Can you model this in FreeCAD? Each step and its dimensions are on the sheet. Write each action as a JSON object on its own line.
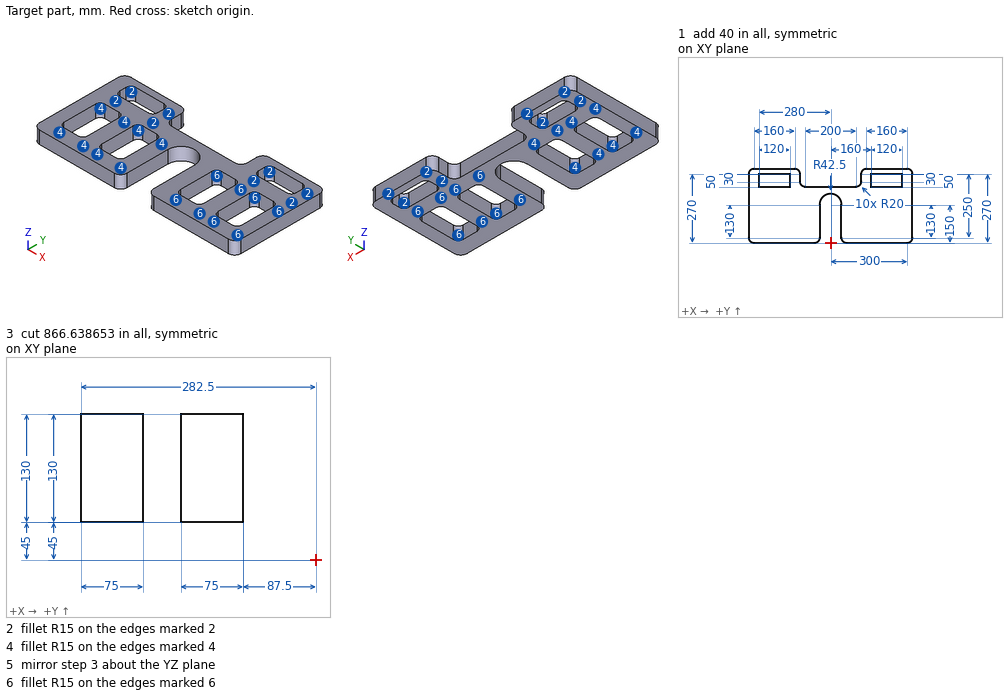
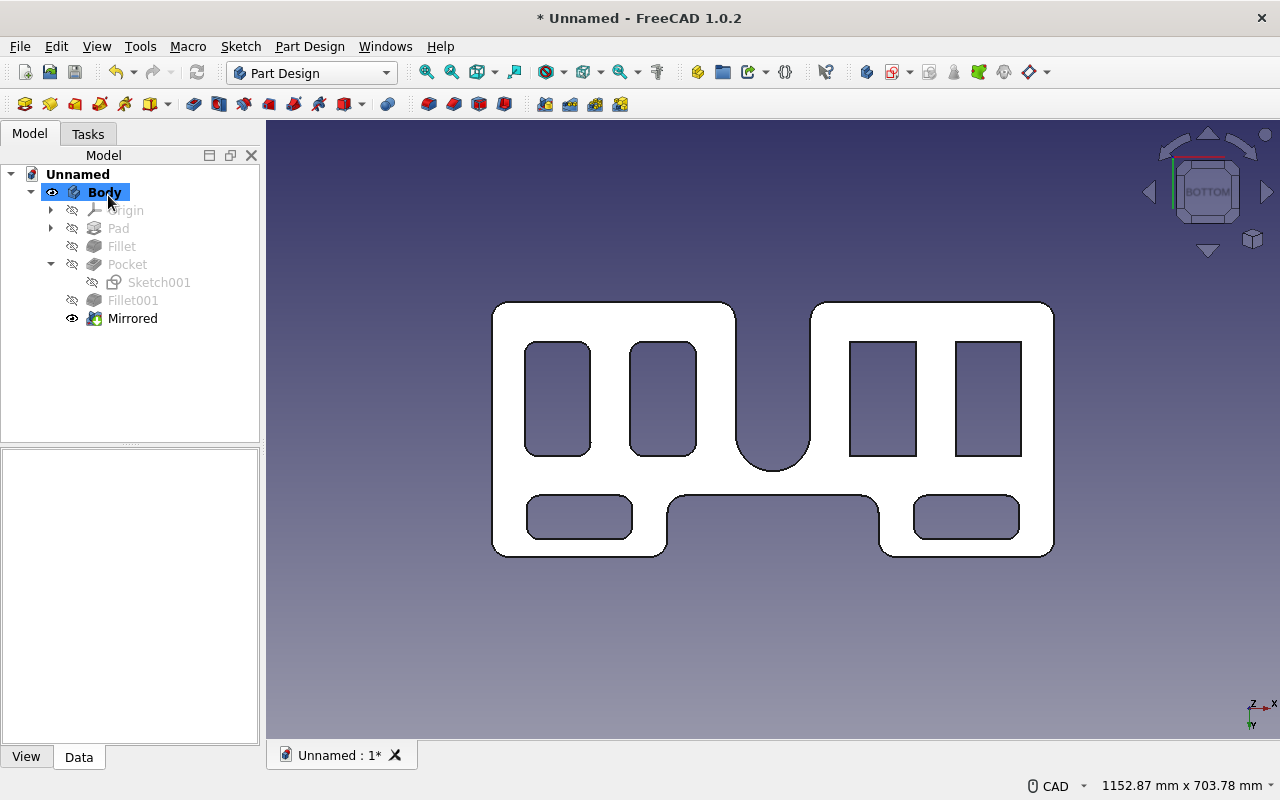
{"action": "key", "text": "4"}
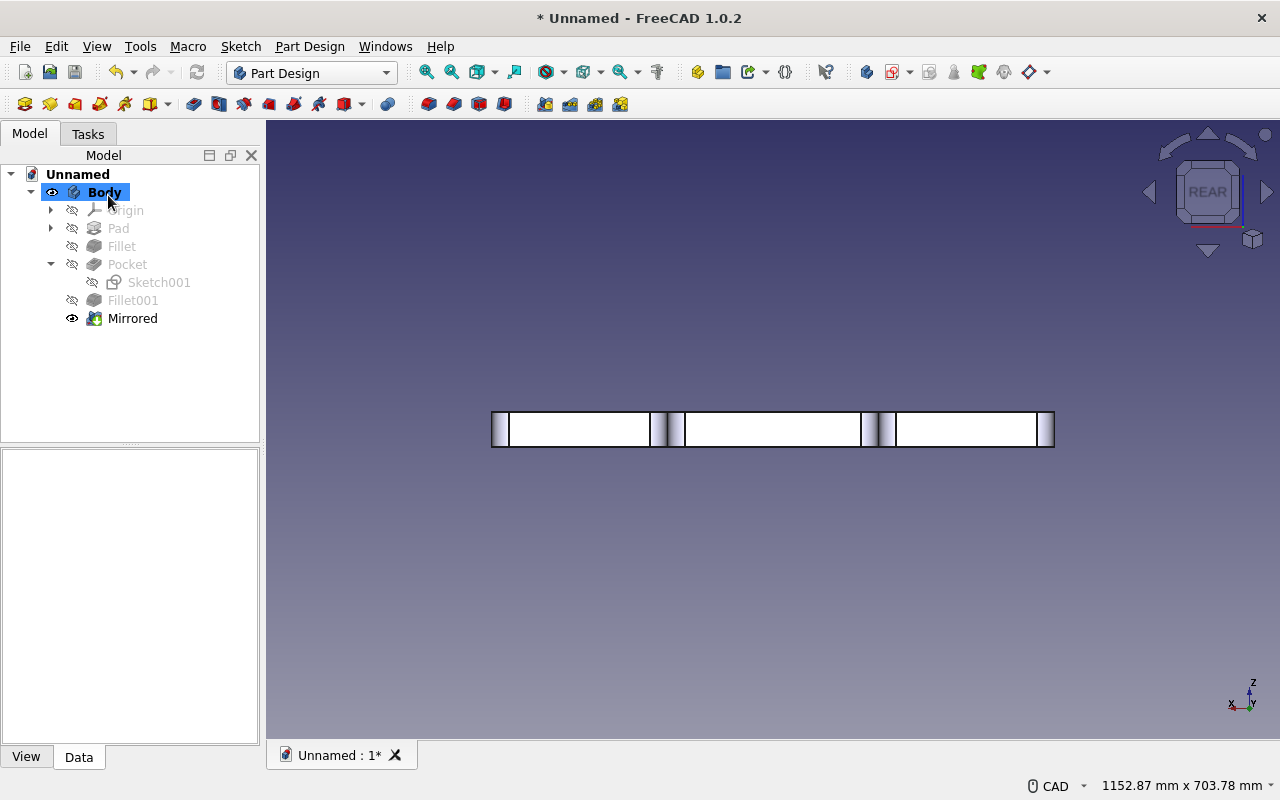
{"action": "key", "text": "6"}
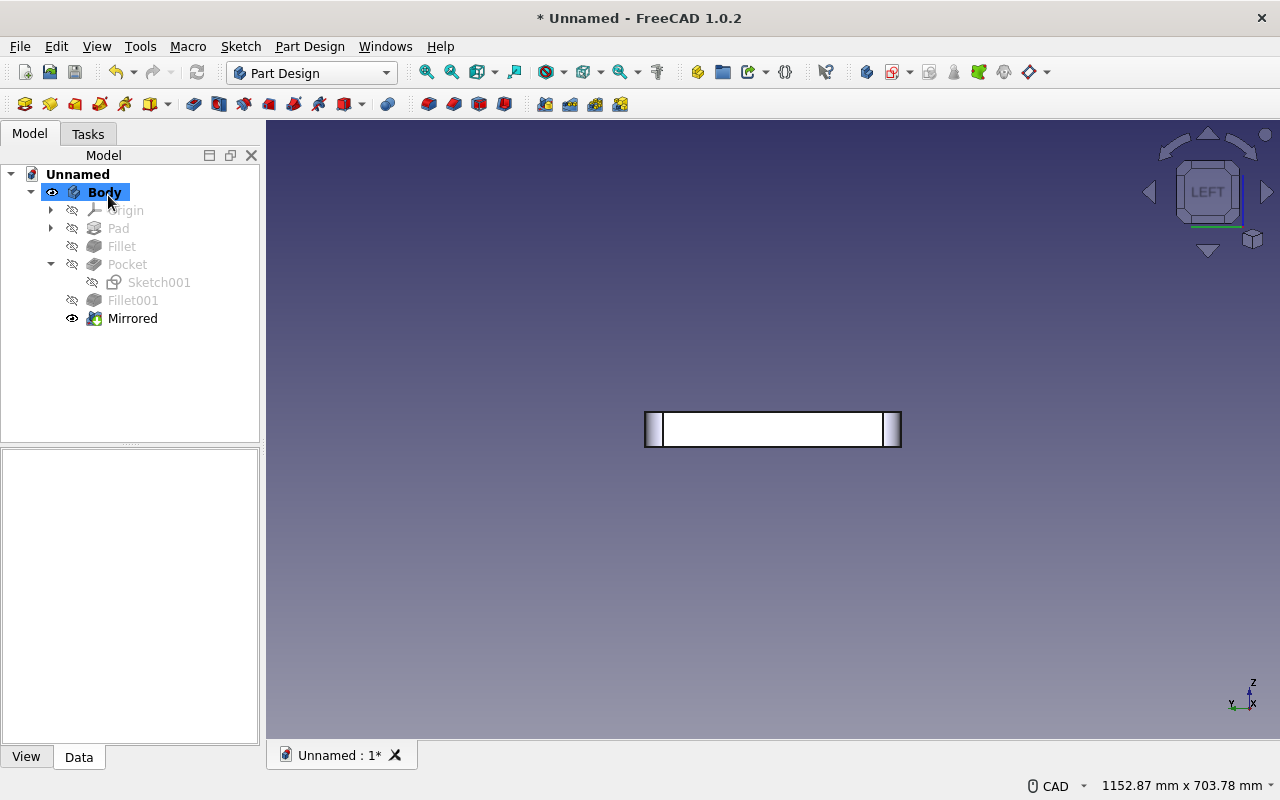
{"action": "left_click", "coordinate": [427, 72]}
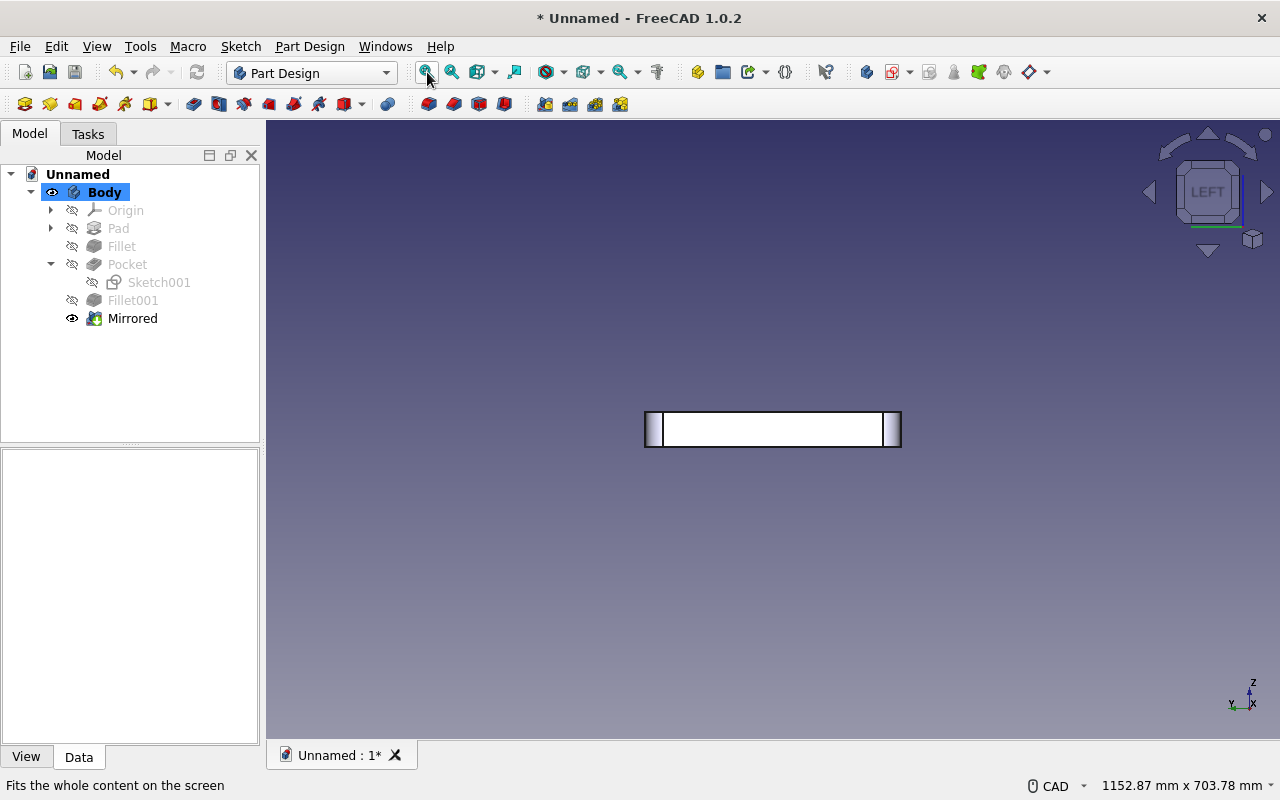
{"action": "key", "text": "v 3"}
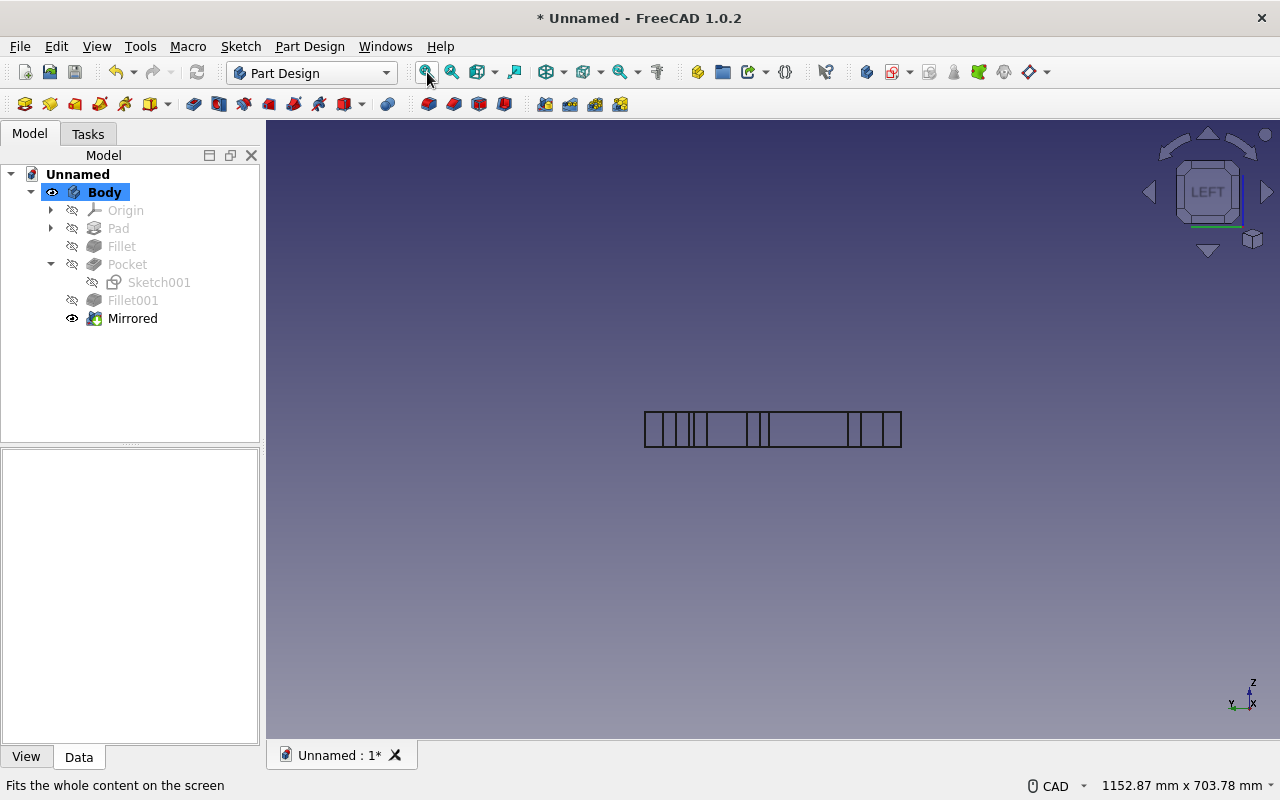
{"action": "key", "text": "0"}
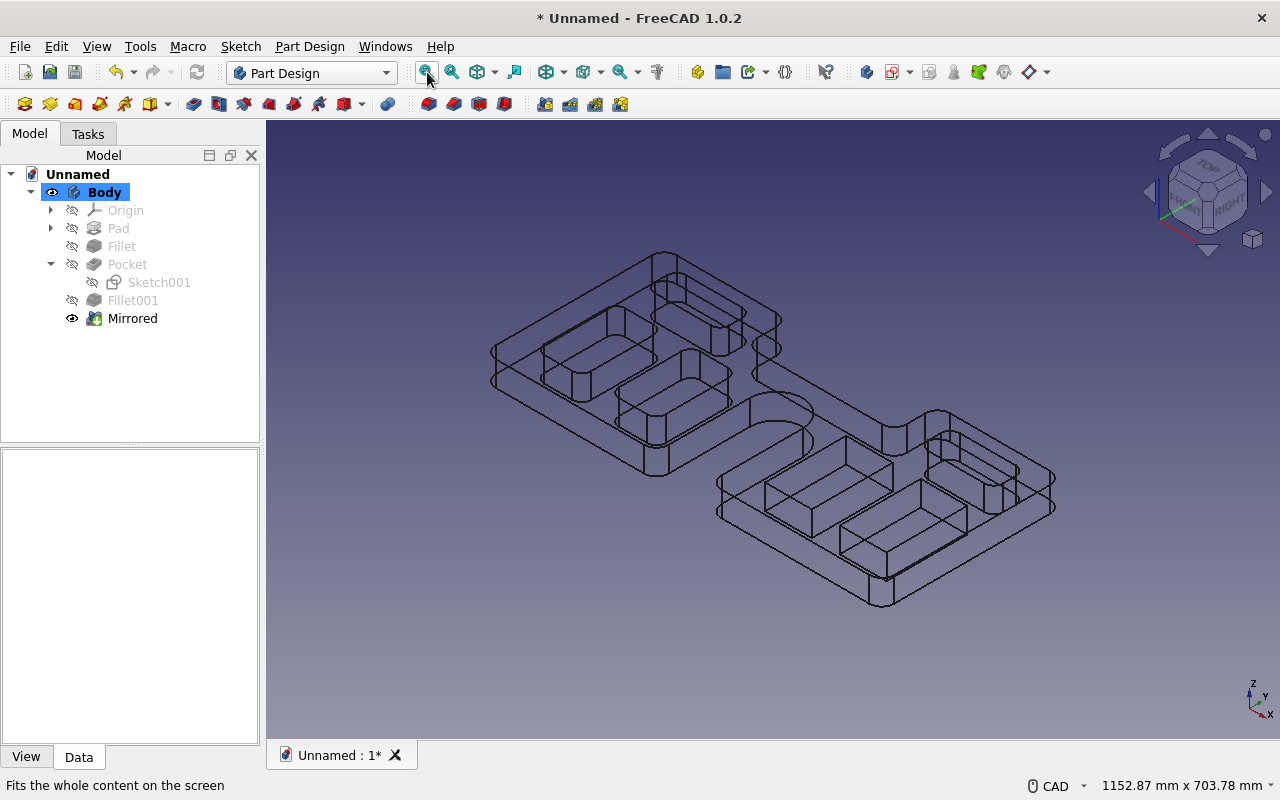
{"action": "left_click", "coordinate": [921, 492]}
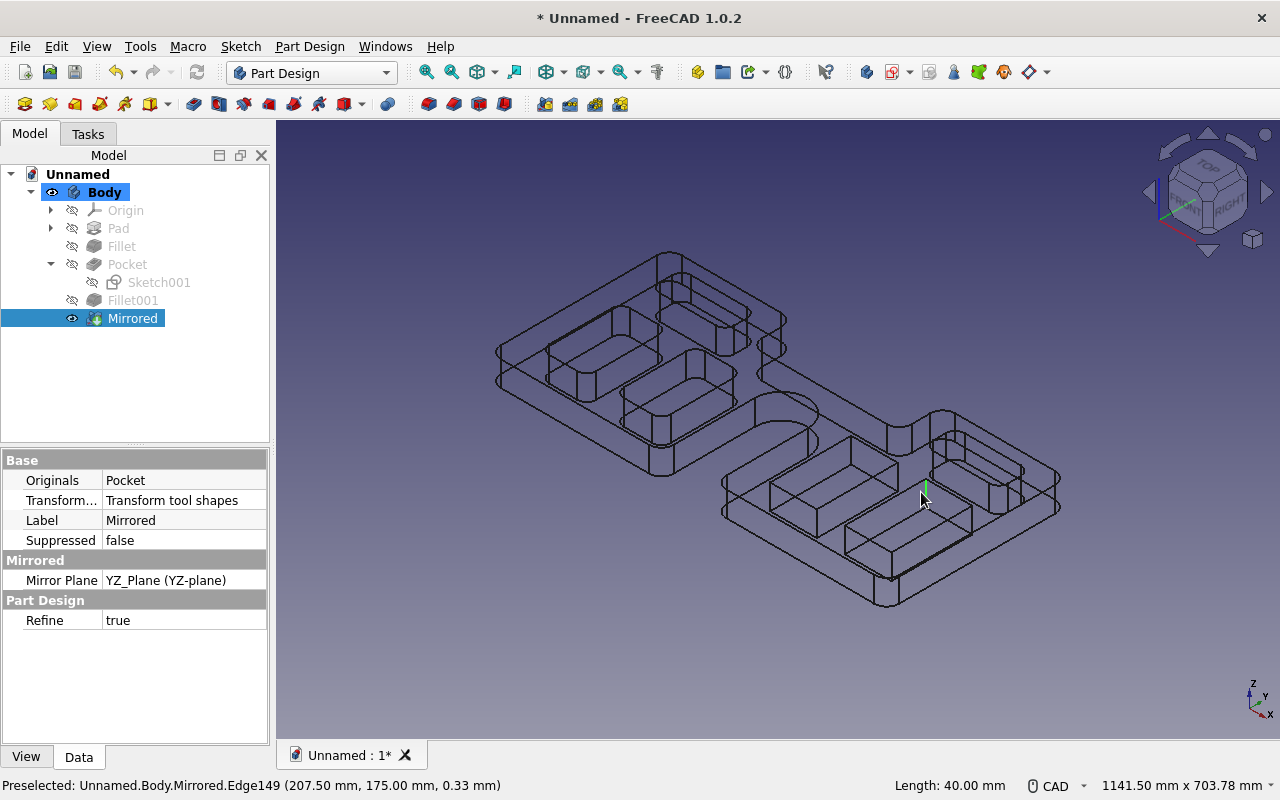
{"action": "left_click", "coordinate": [845, 539], "text": "ctrl"}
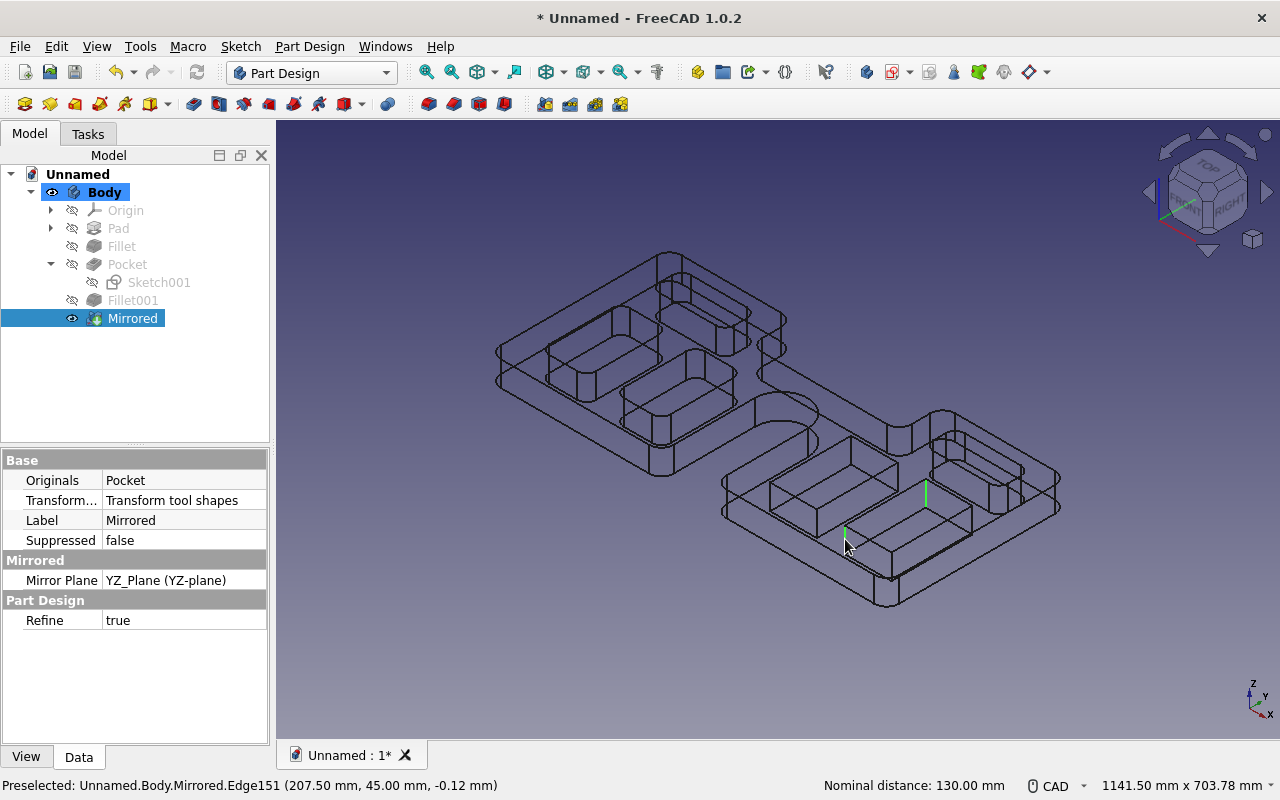
{"action": "left_click", "coordinate": [892, 566], "text": "ctrl"}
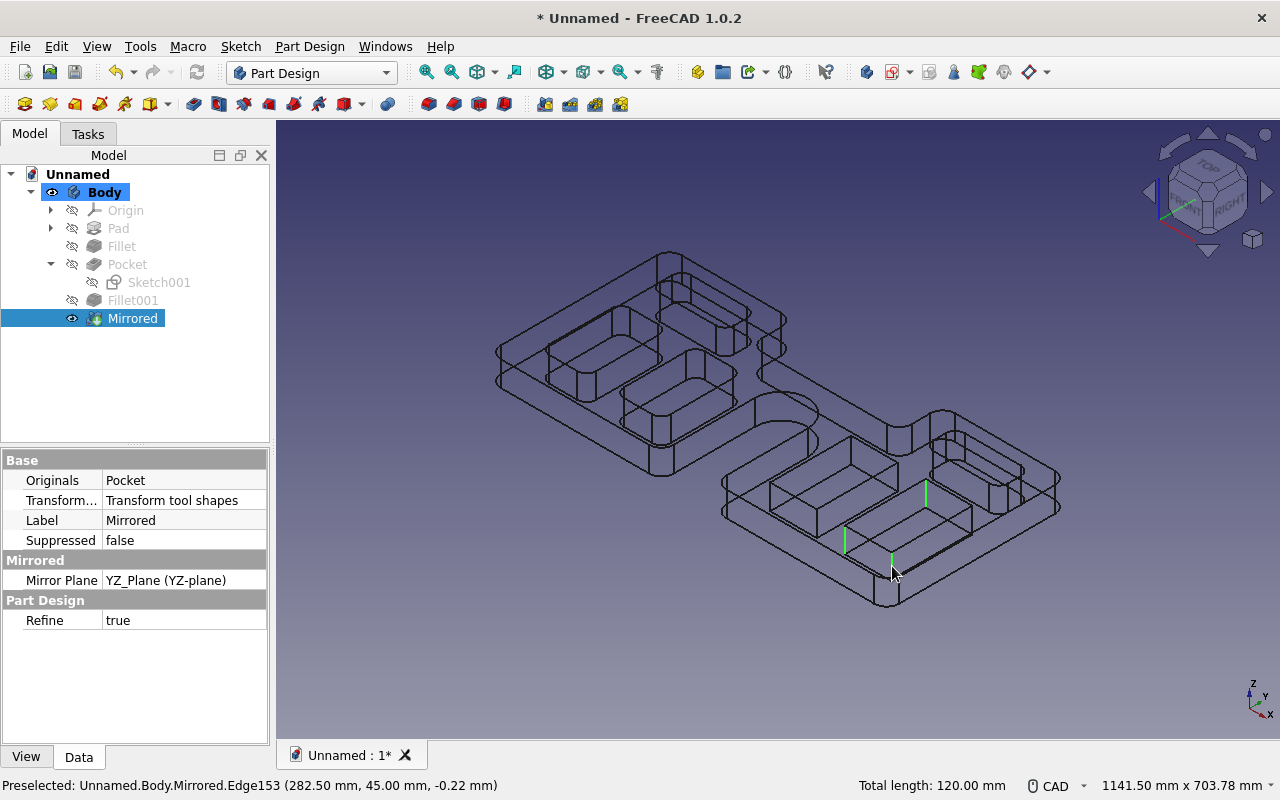
{"action": "left_click", "coordinate": [972, 519], "text": "ctrl"}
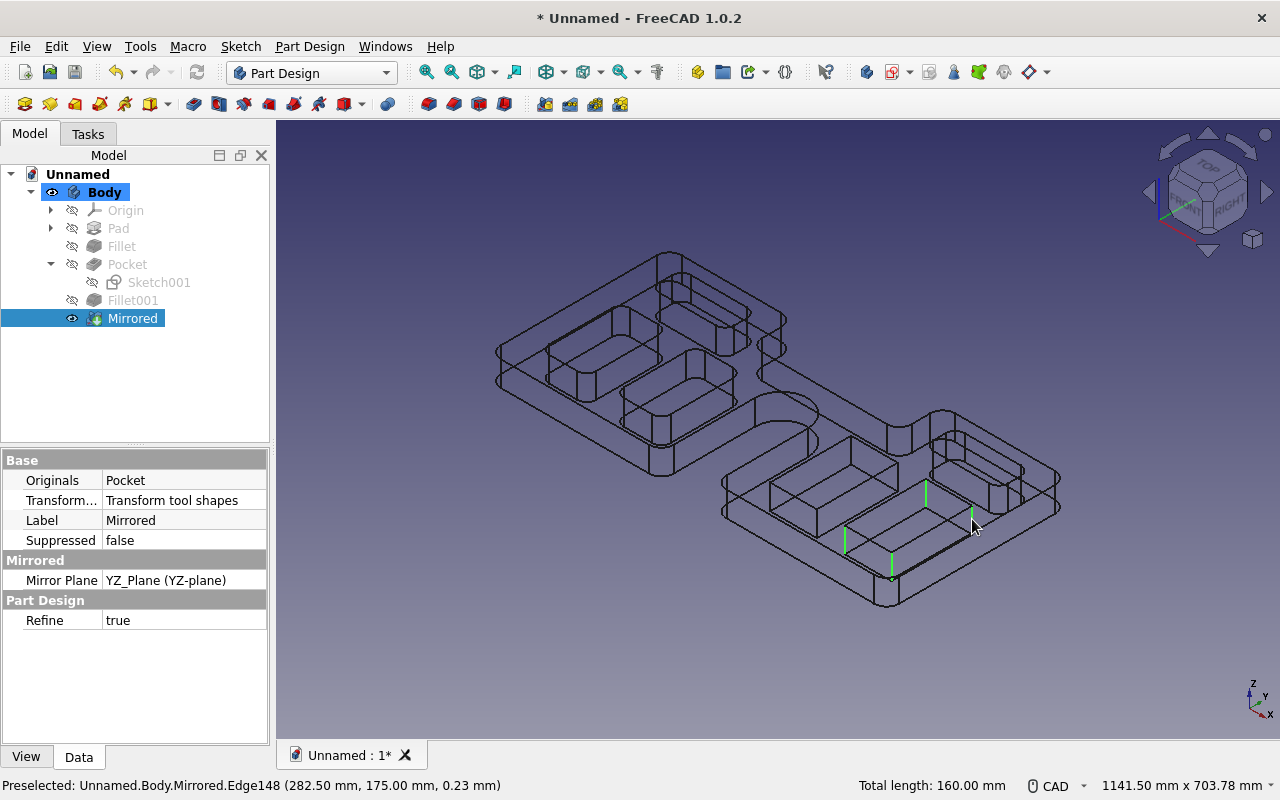
{"action": "left_click", "coordinate": [851, 449], "text": "ctrl"}